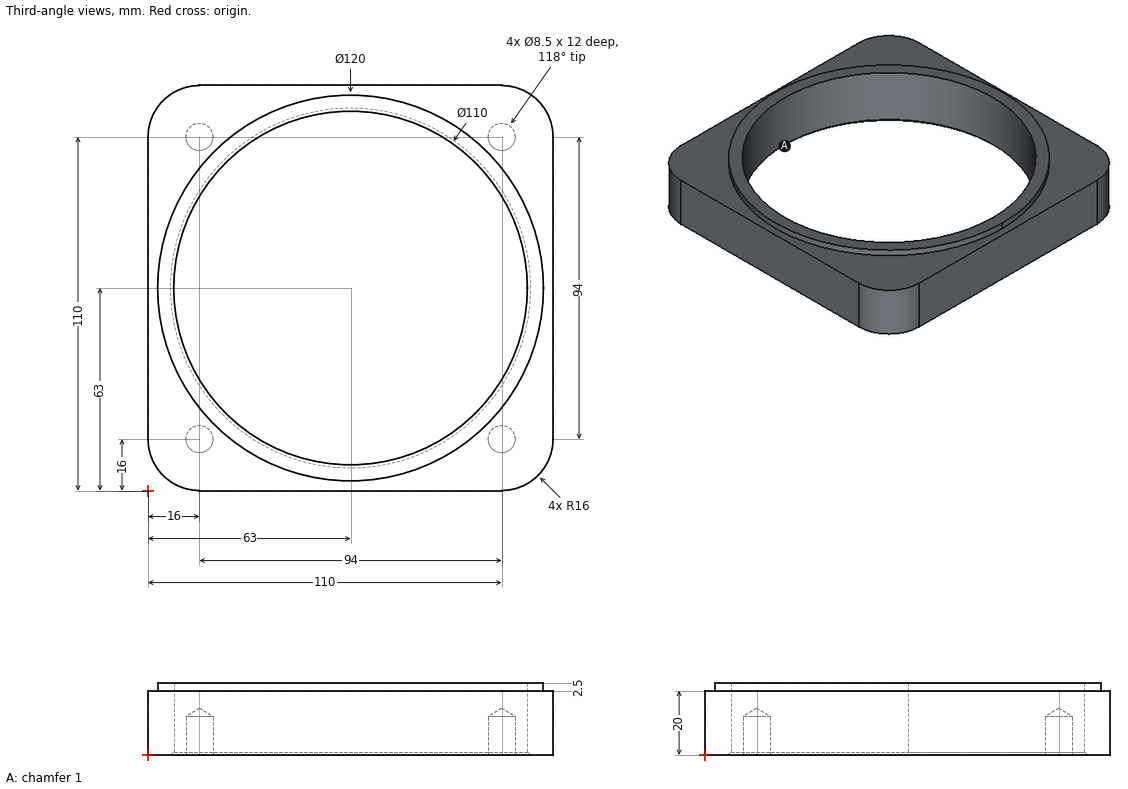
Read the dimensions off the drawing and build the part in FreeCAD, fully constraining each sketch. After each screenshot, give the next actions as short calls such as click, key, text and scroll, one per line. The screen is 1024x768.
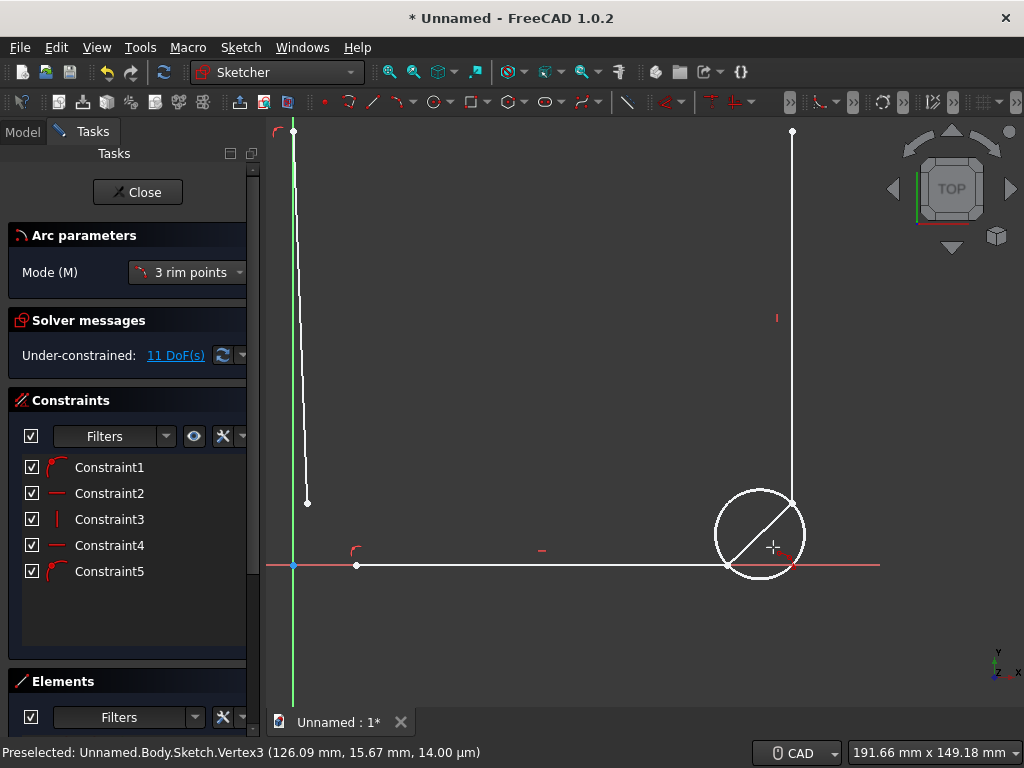
click(773, 547)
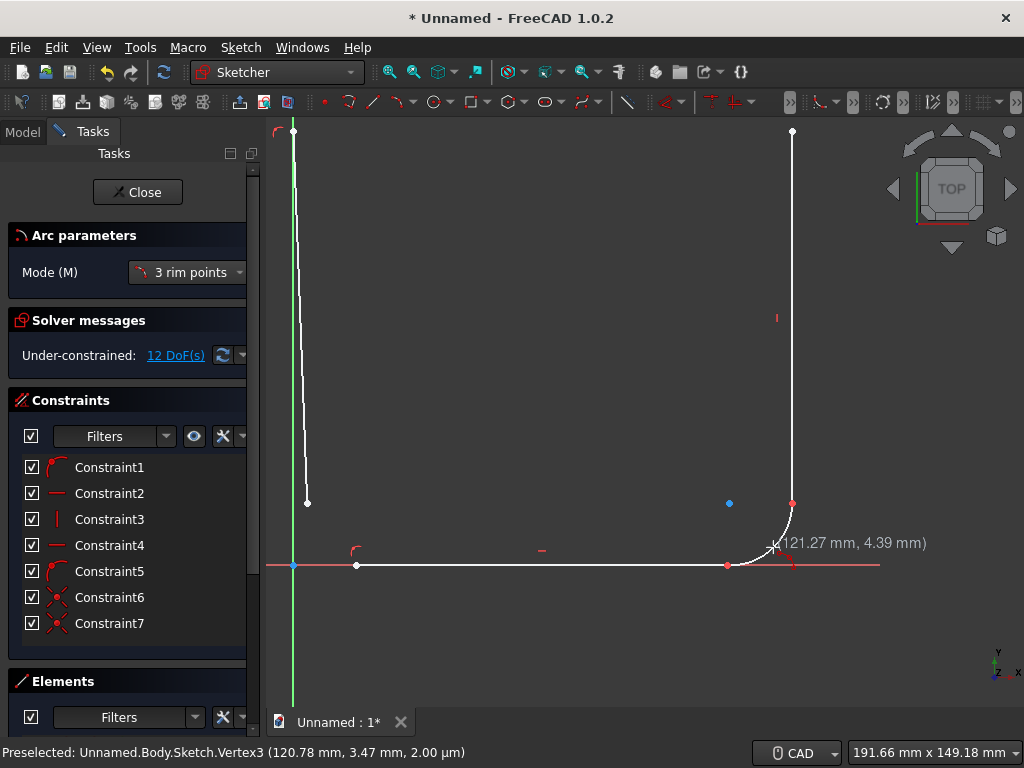
scroll(730, 679, down, 1)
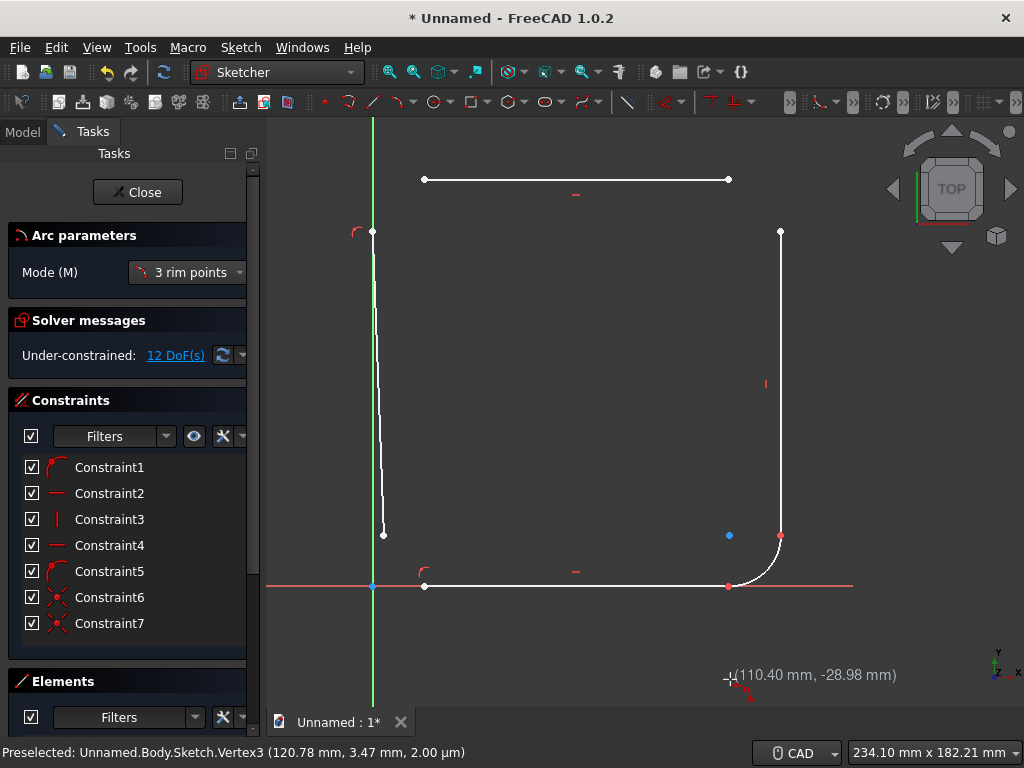
click(781, 231)
click(728, 180)
click(765, 193)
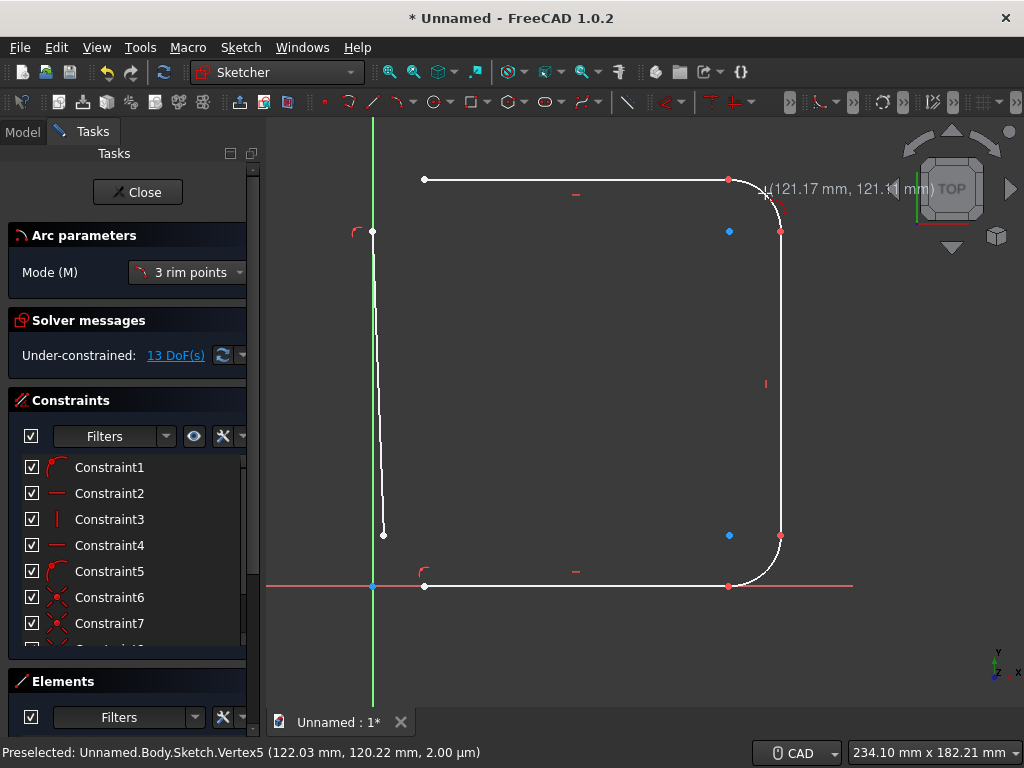
click(424, 180)
click(373, 231)
click(388, 193)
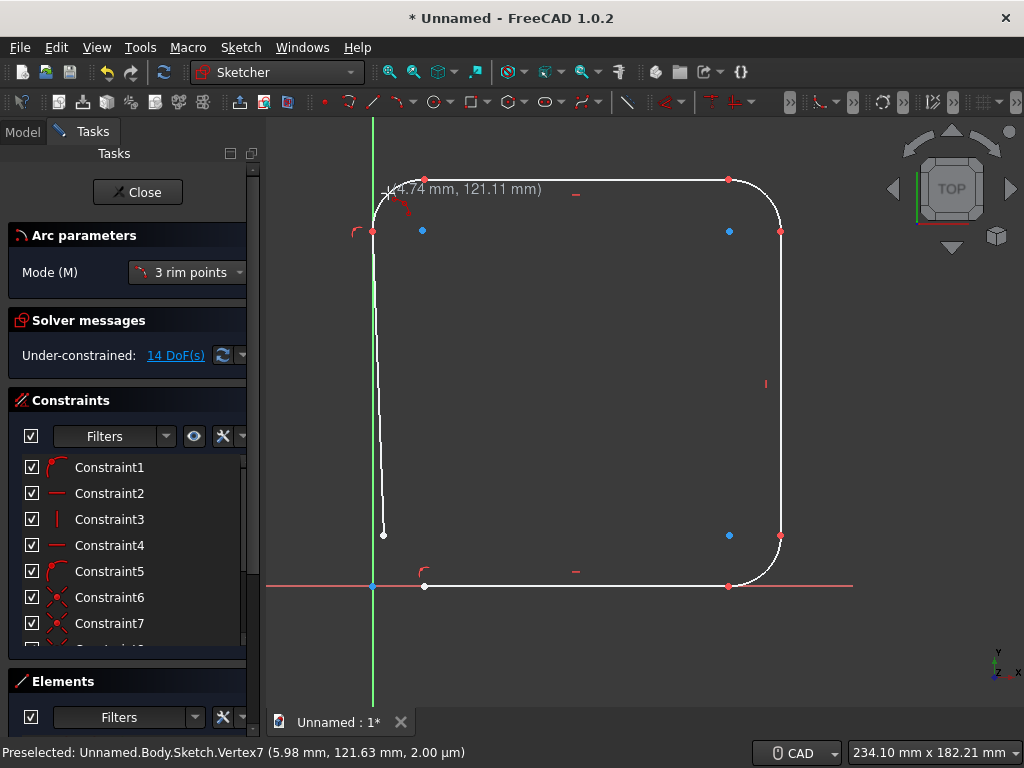
click(384, 535)
click(424, 586)
click(388, 571)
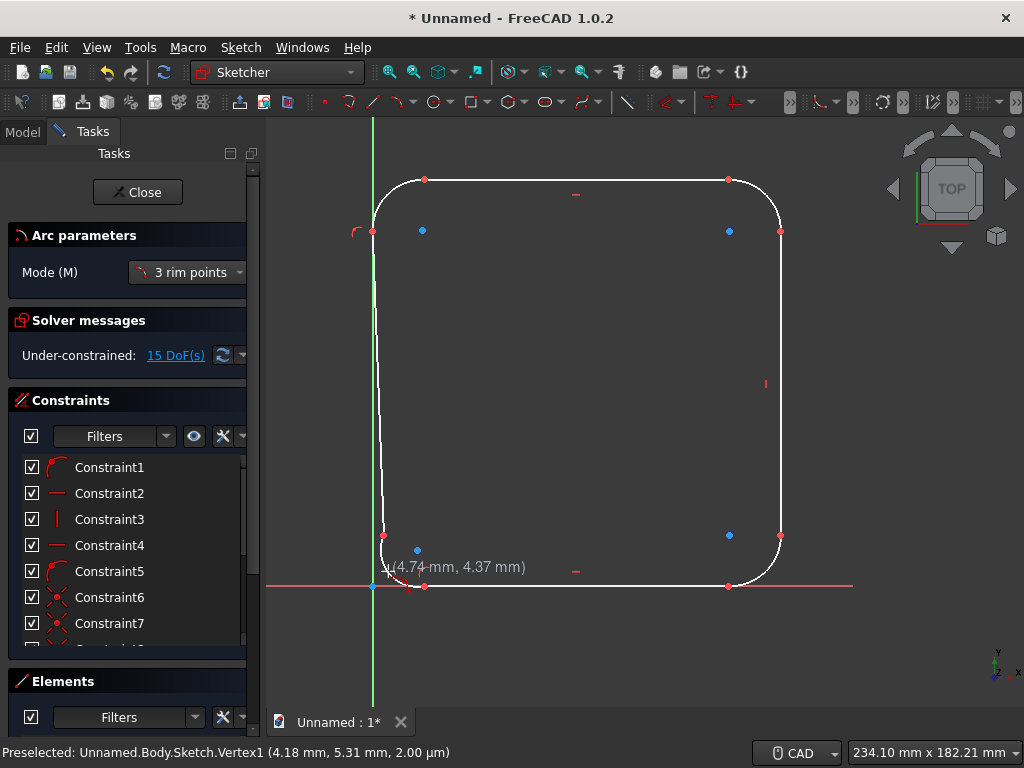
click(434, 102)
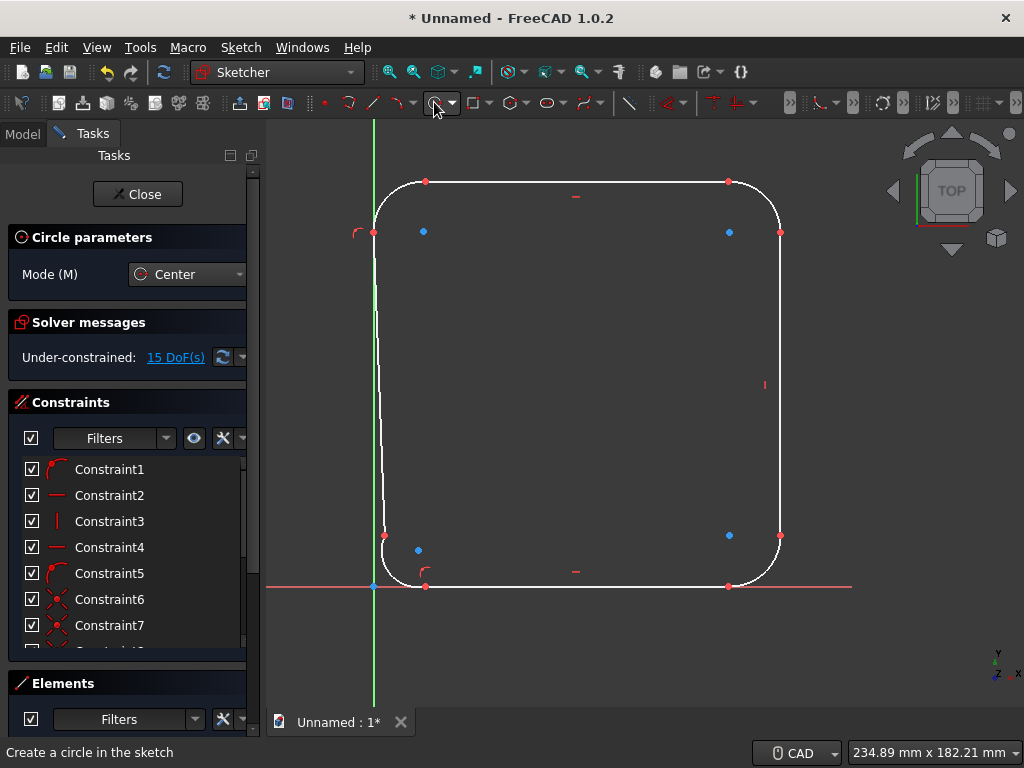
click(577, 383)
move(702, 258)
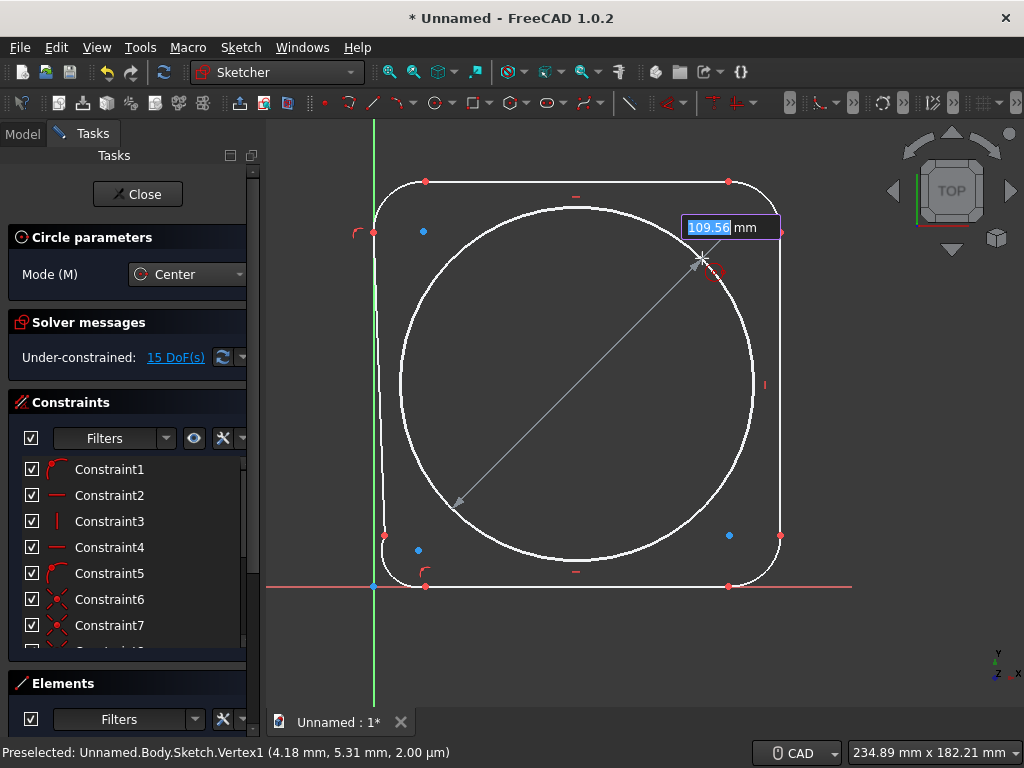
text(110)
key(Return)
key(Escape)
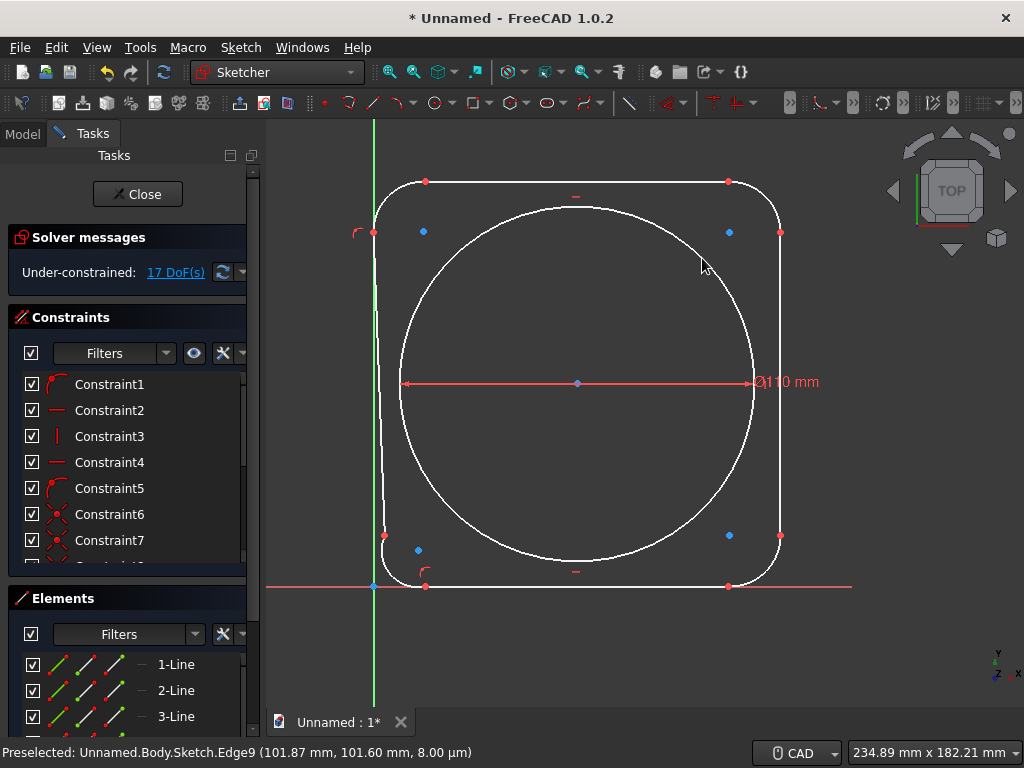
click(516, 587)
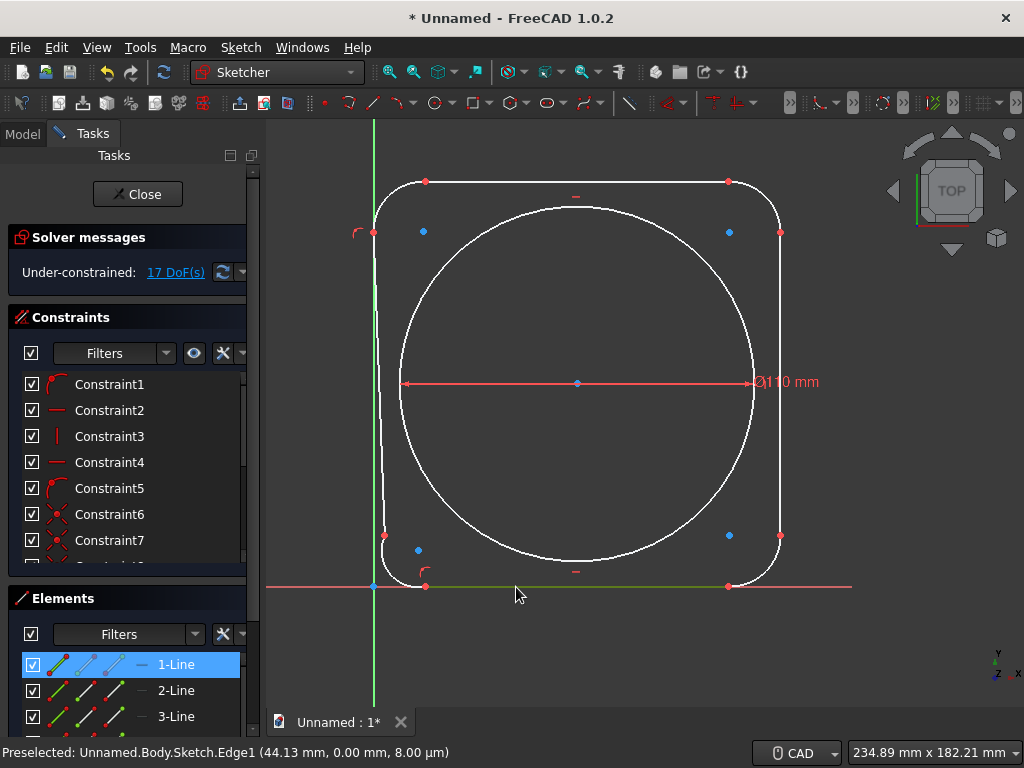
click(775, 559)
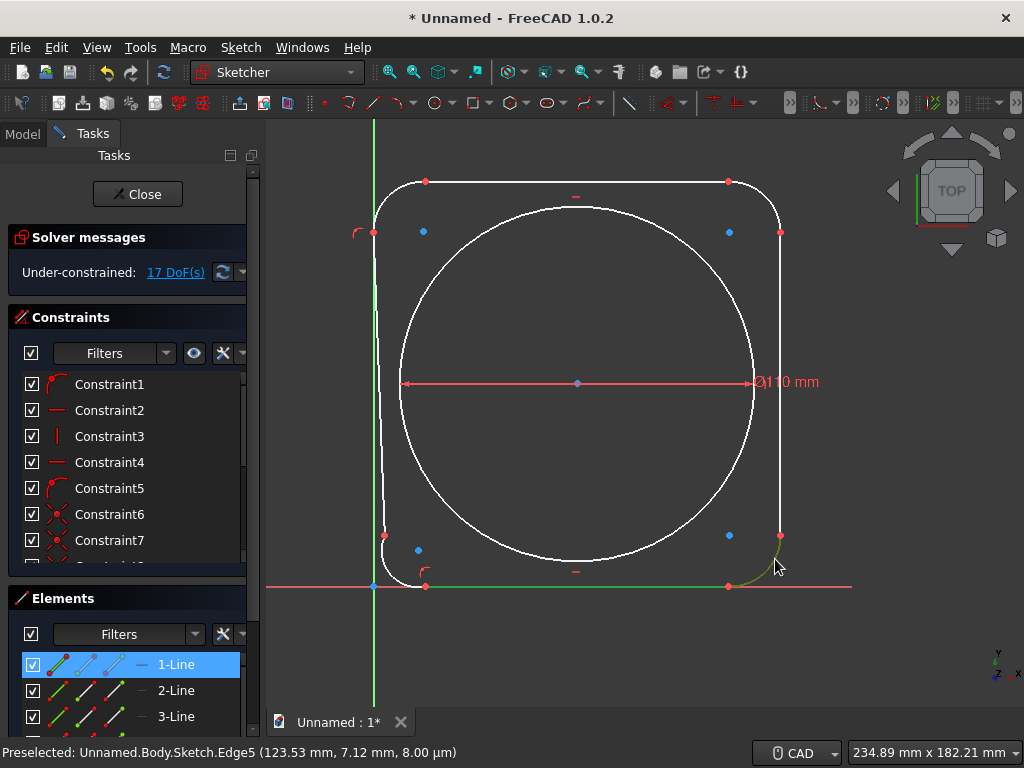
key(t)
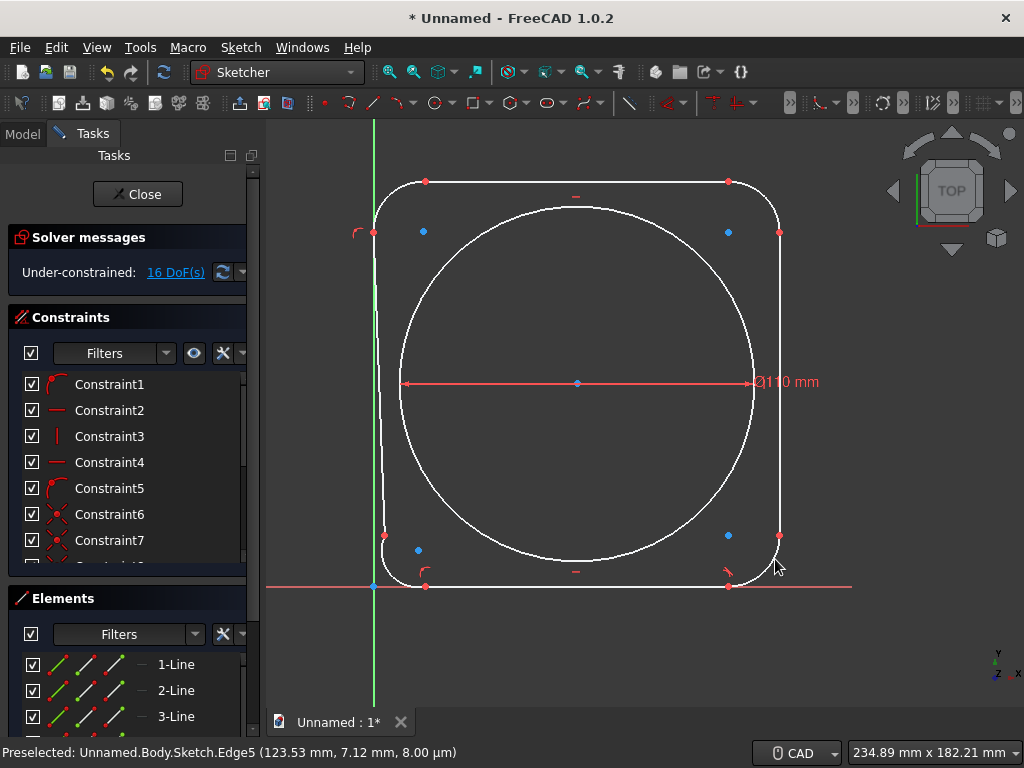
click(516, 587)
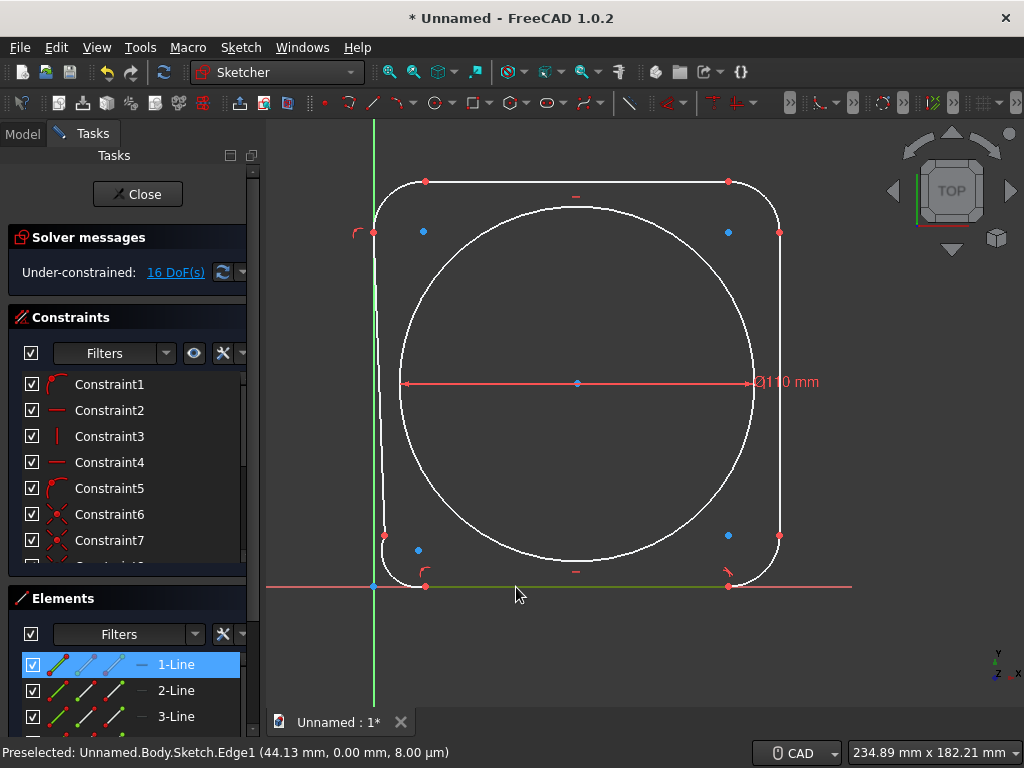
scroll(383, 559, up, 3)